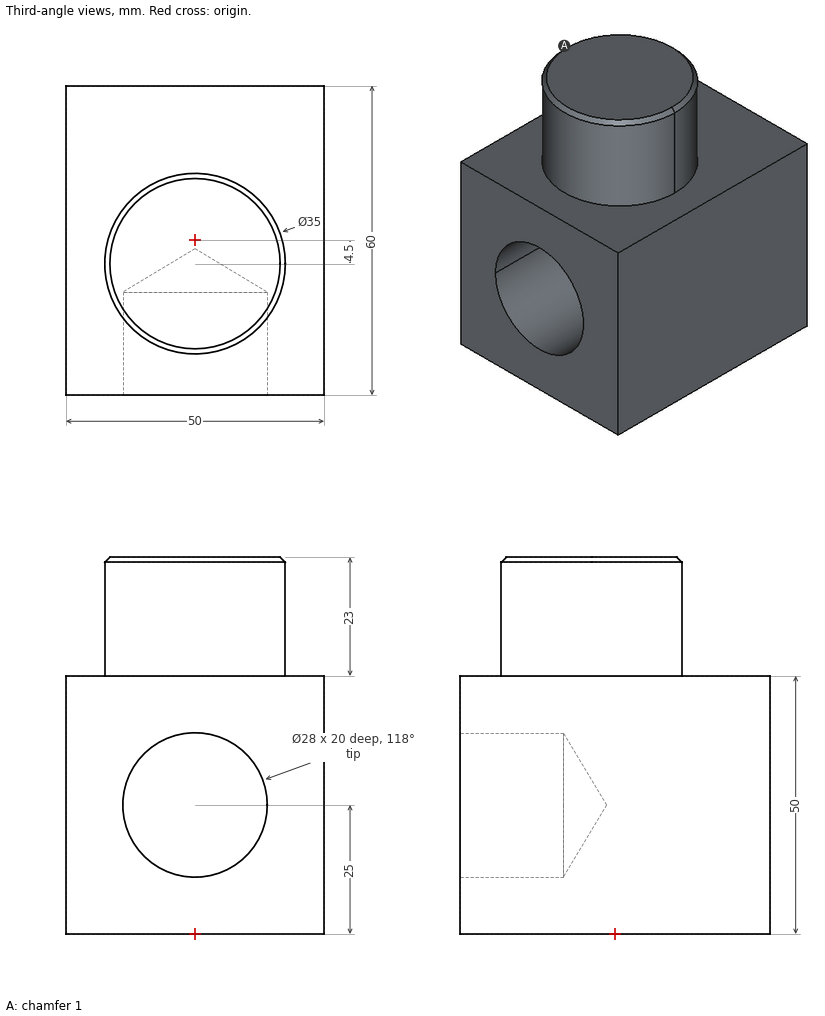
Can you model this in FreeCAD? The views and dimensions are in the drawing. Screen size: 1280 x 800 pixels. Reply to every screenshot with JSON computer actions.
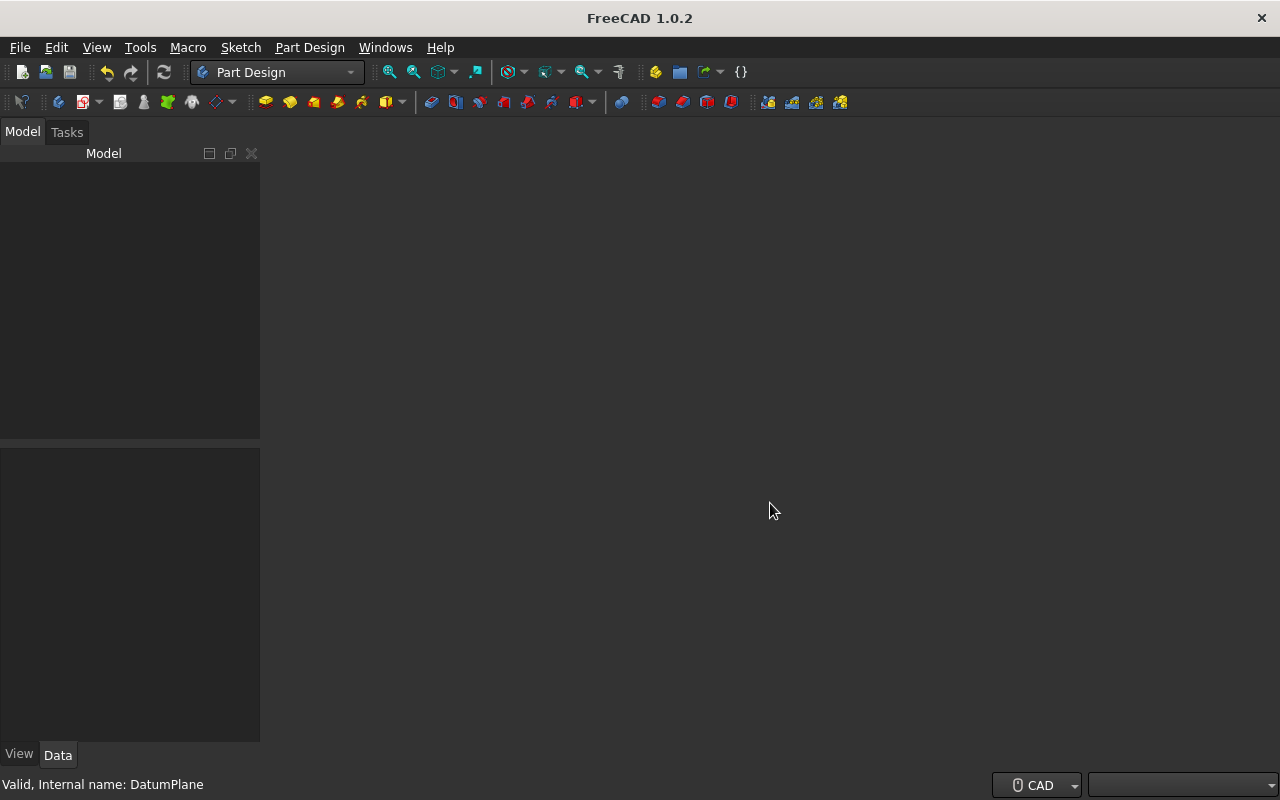
{"action": "left_click", "coordinate": [22, 72]}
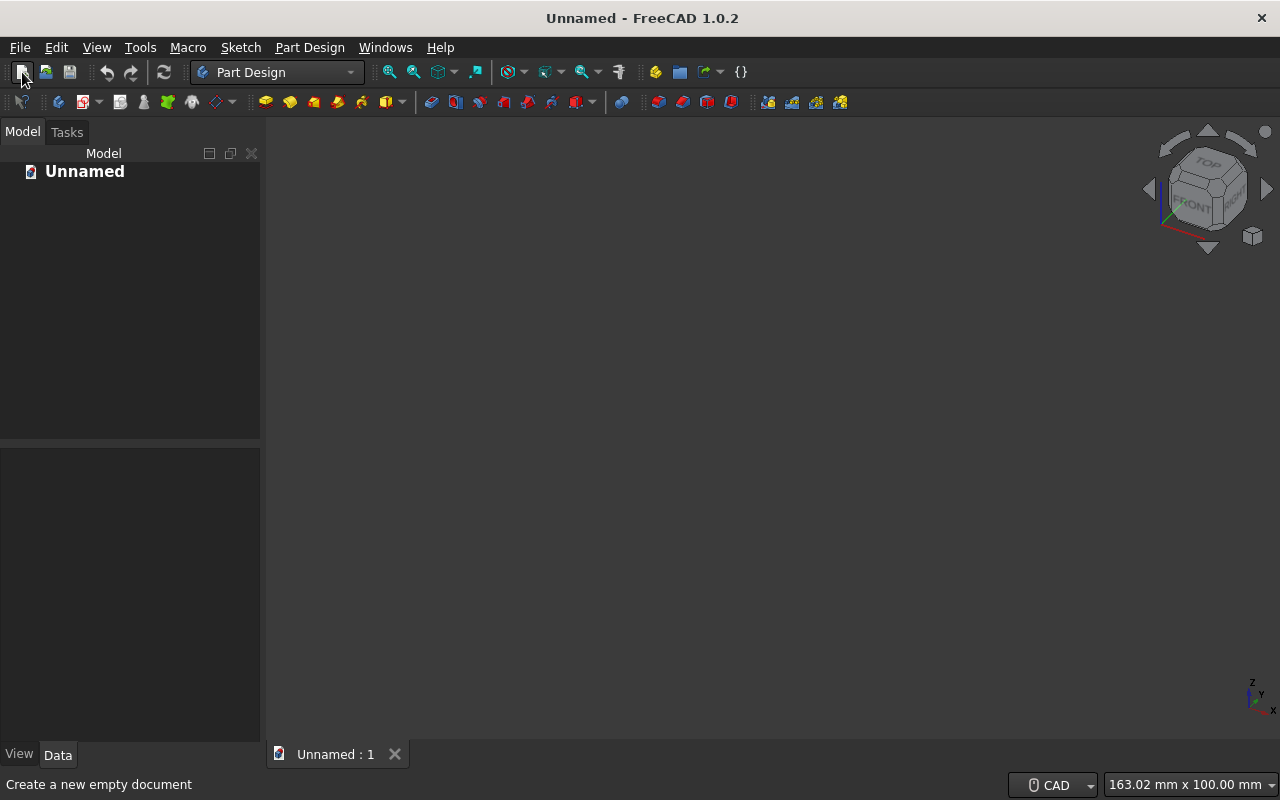
{"action": "left_click", "coordinate": [84, 102]}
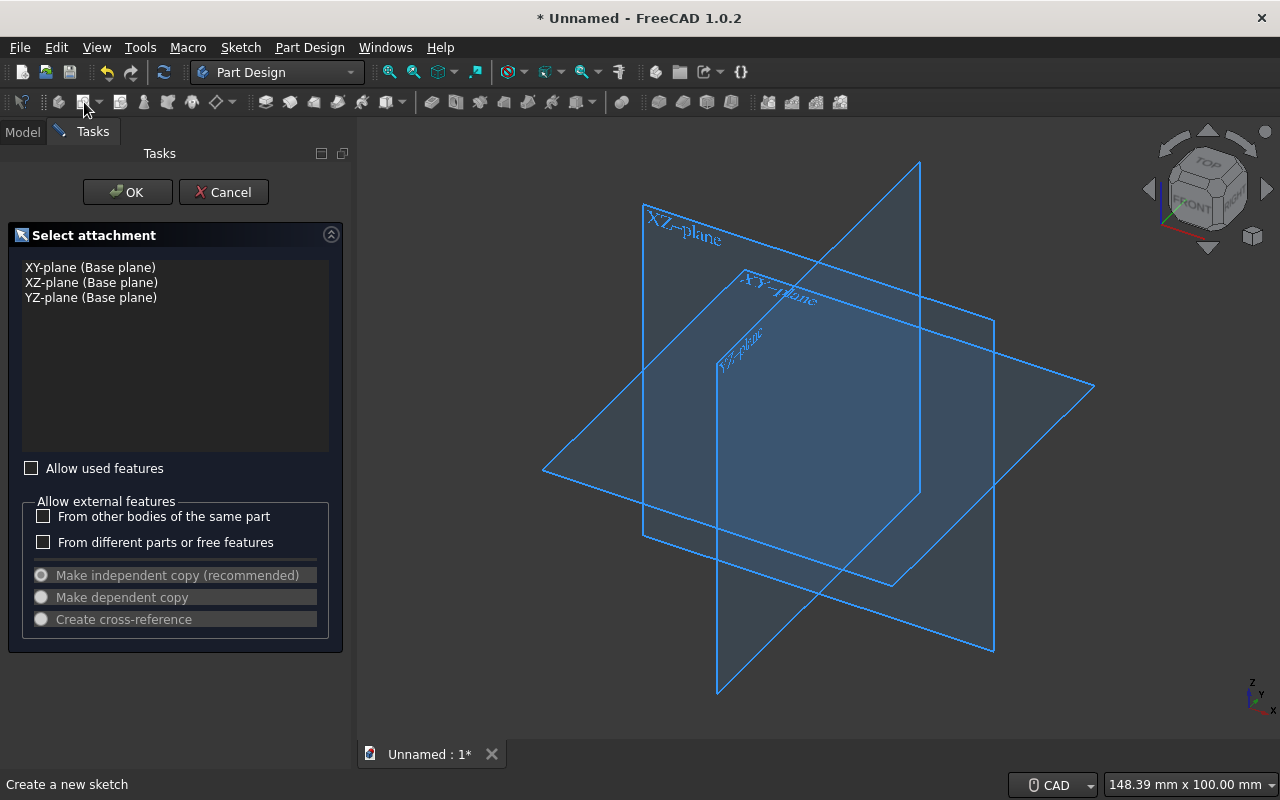
{"action": "left_click", "coordinate": [82, 268]}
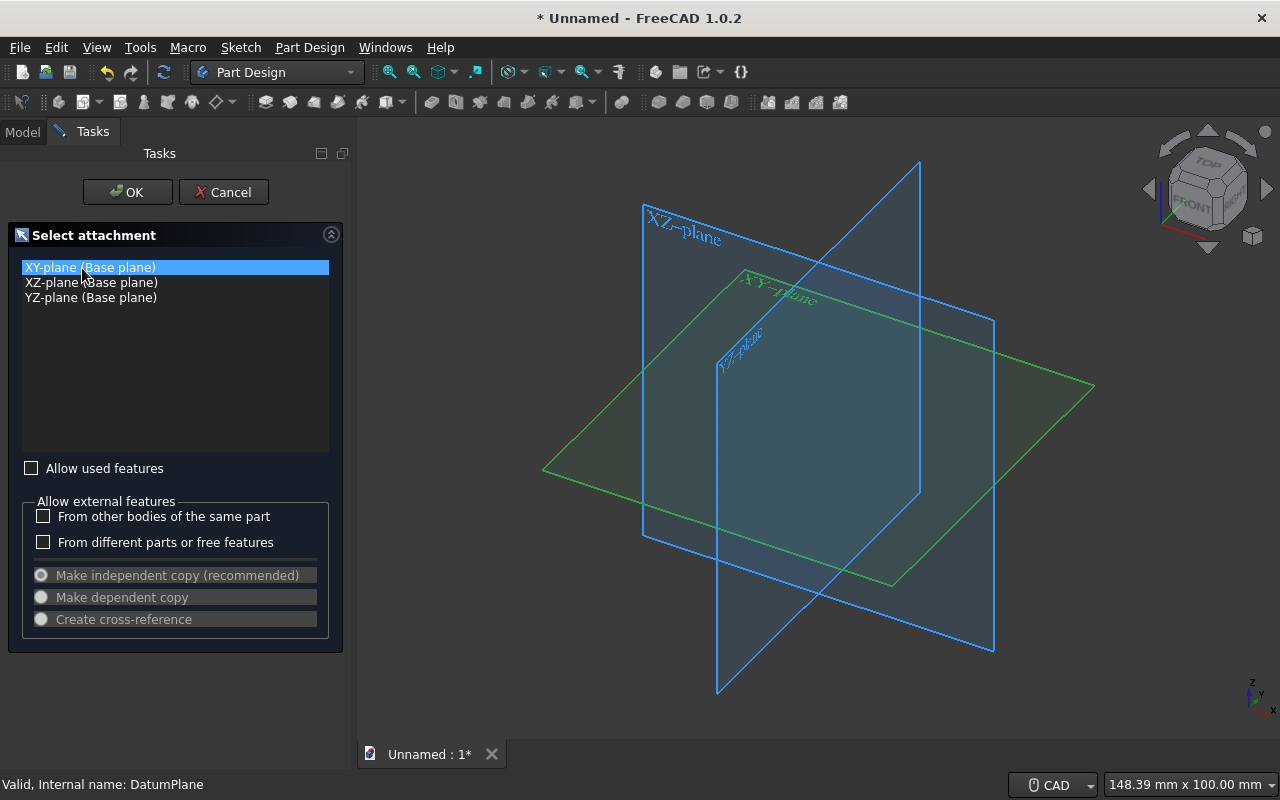
{"action": "left_click", "coordinate": [128, 192]}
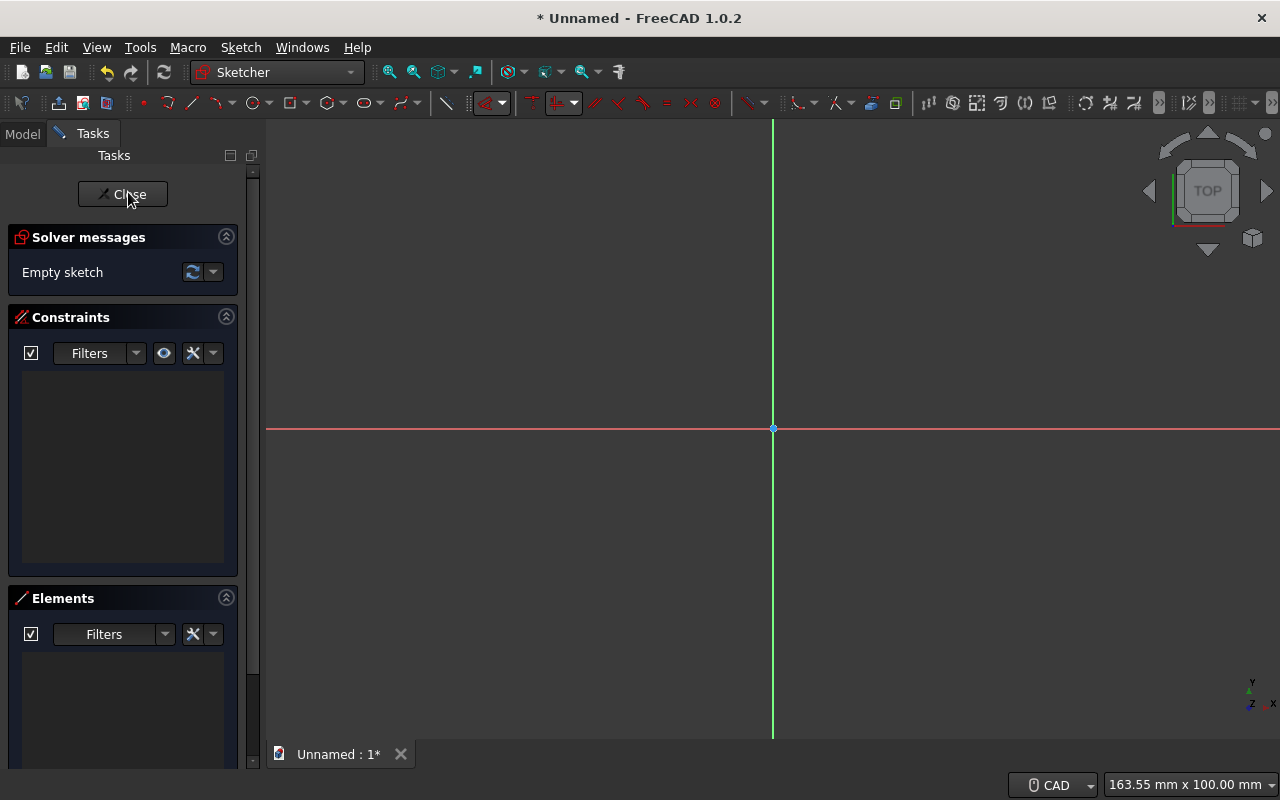
{"action": "left_click", "coordinate": [290, 104]}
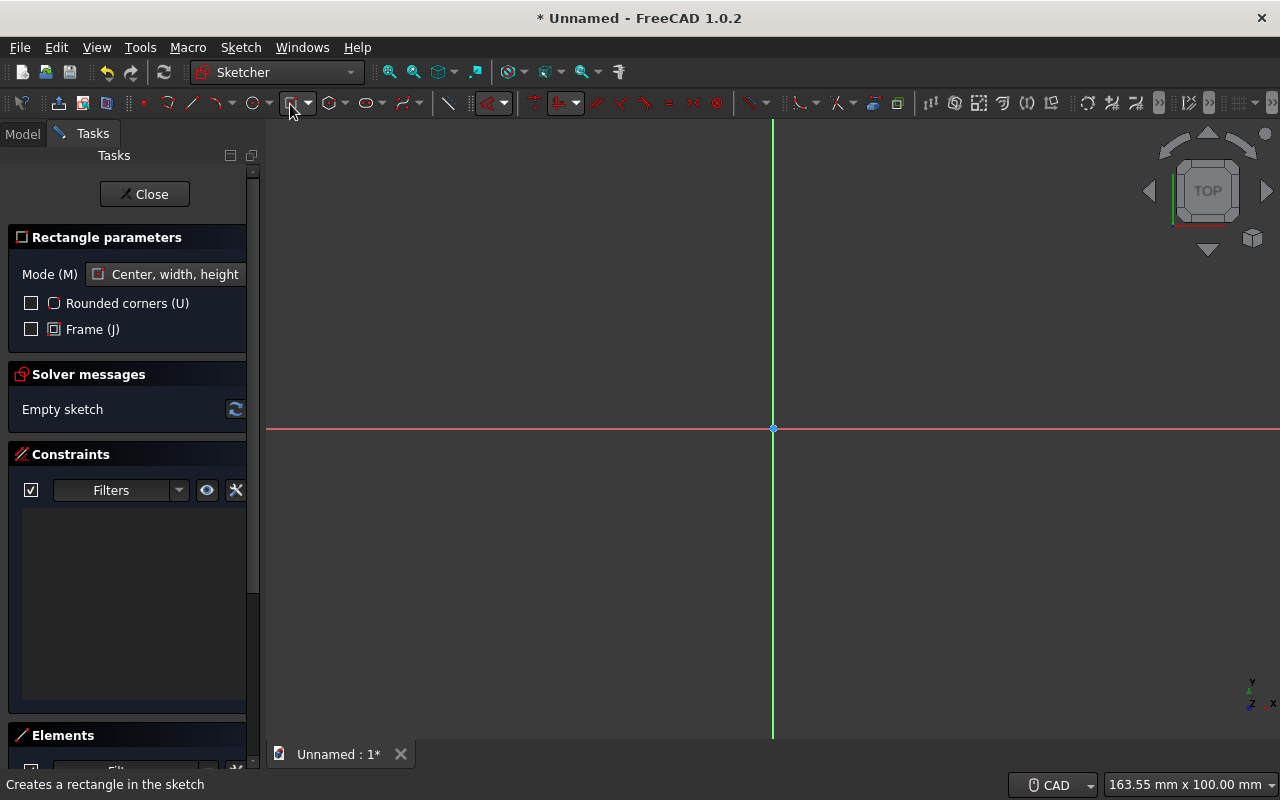
{"action": "left_click", "coordinate": [773, 429]}
{"action": "mouse_move", "coordinate": [928, 243]}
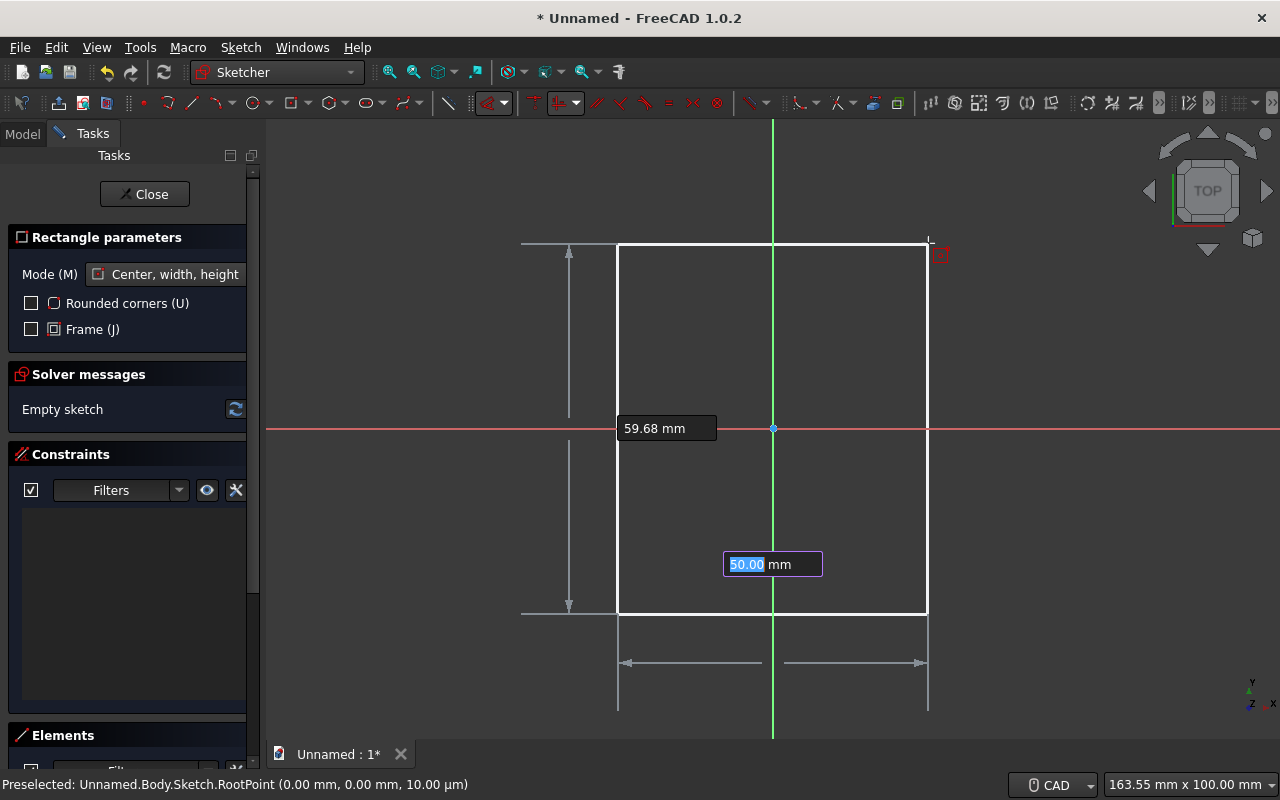
{"action": "type", "text": "50"}
{"action": "key", "text": "Tab"}
{"action": "type", "text": "60"}
{"action": "key", "text": "Return"}
{"action": "key", "text": "Escape"}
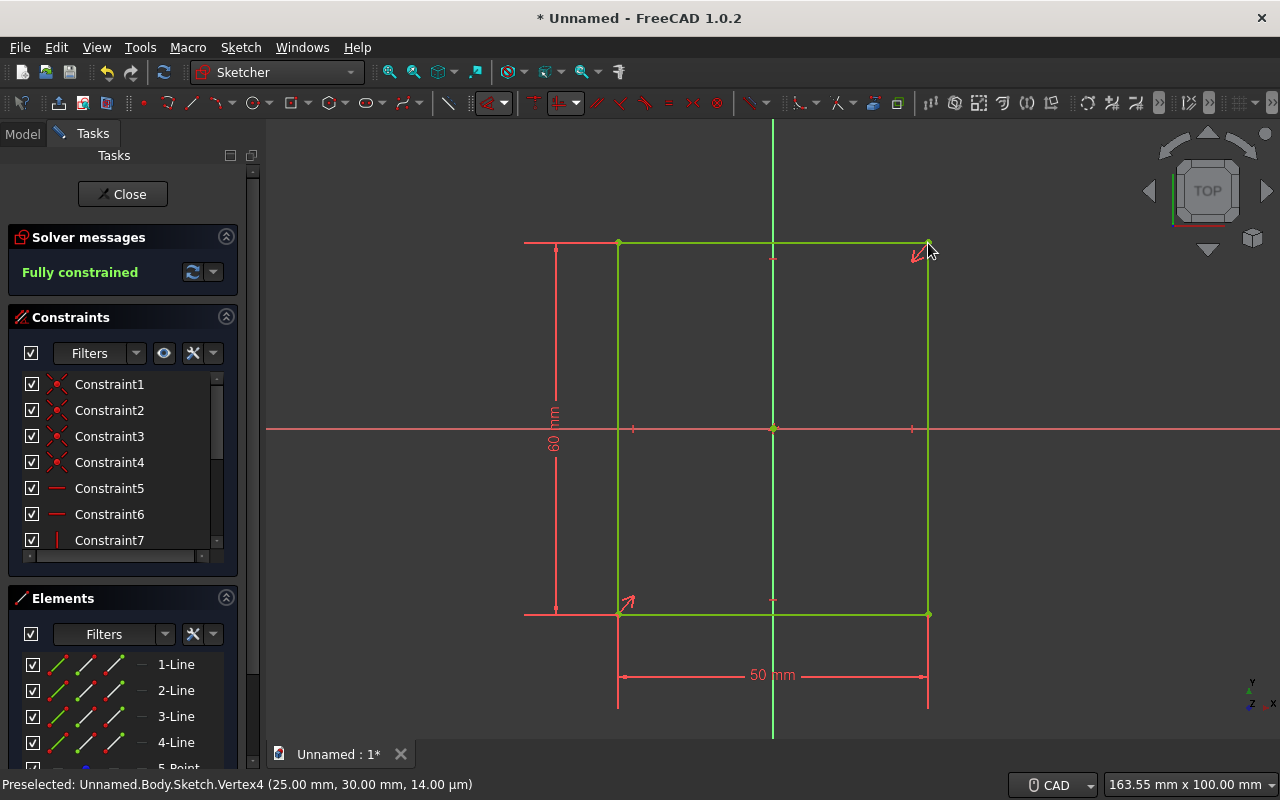
{"action": "left_click", "coordinate": [123, 194]}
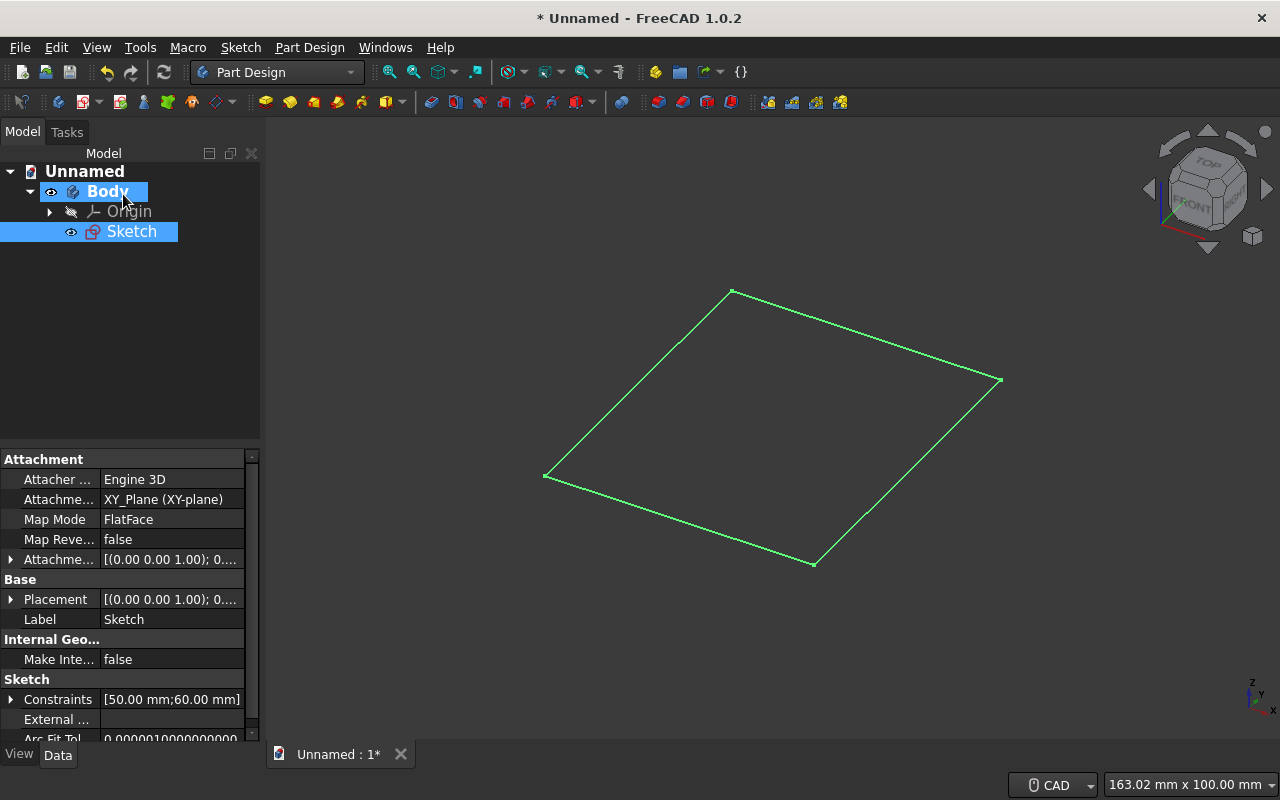
{"action": "left_click", "coordinate": [266, 102]}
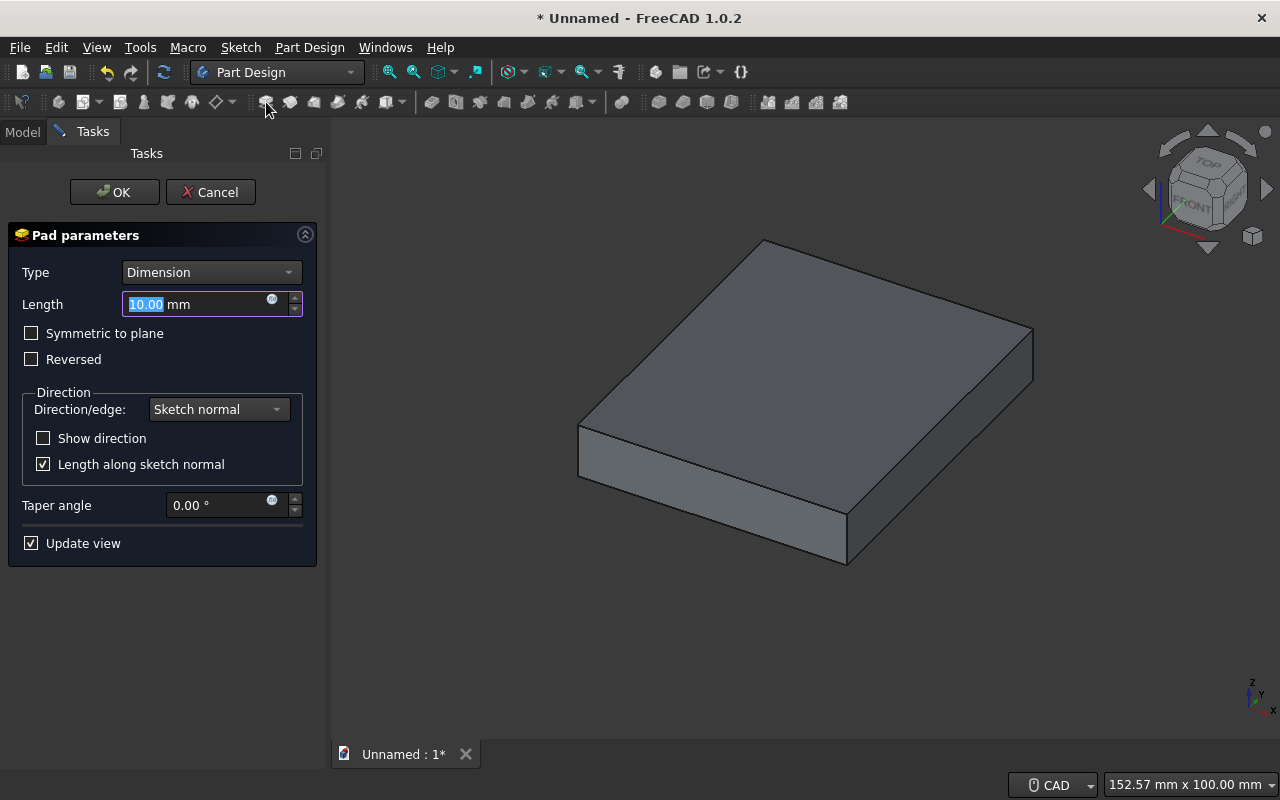
{"action": "type", "text": "50"}
{"action": "key", "text": "Tab"}